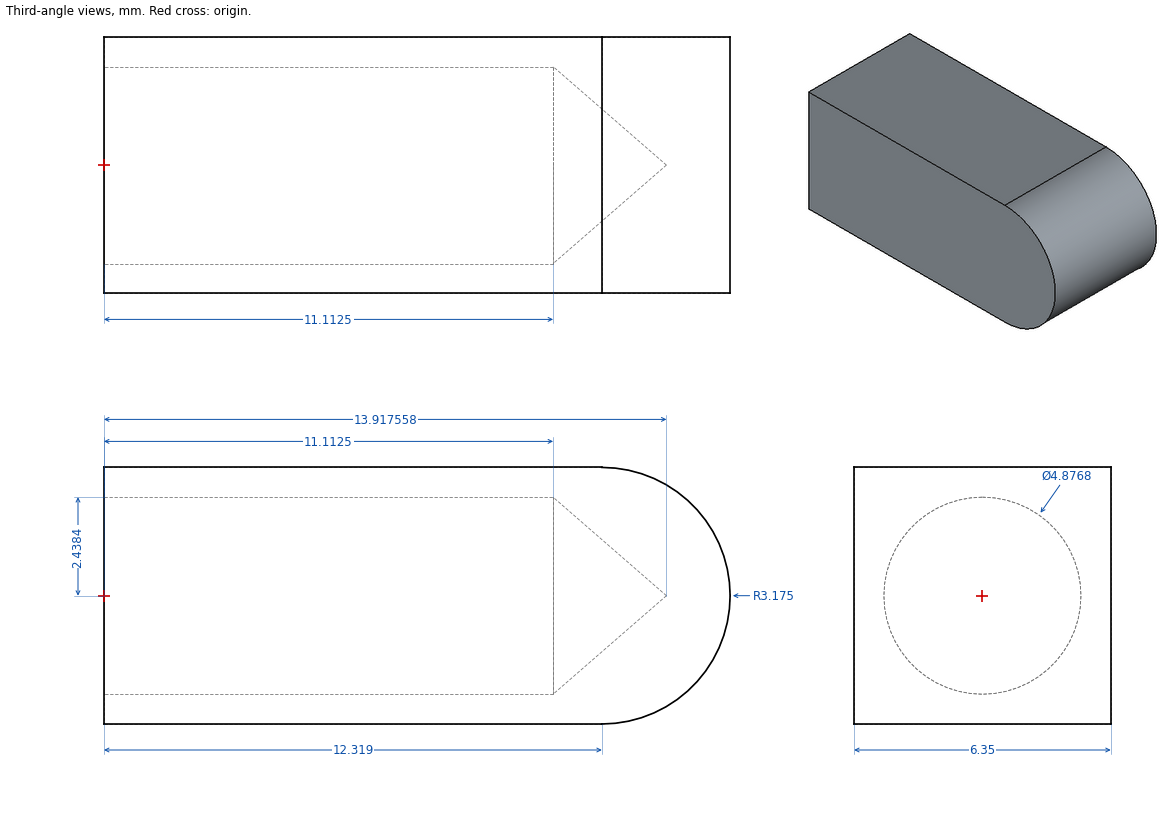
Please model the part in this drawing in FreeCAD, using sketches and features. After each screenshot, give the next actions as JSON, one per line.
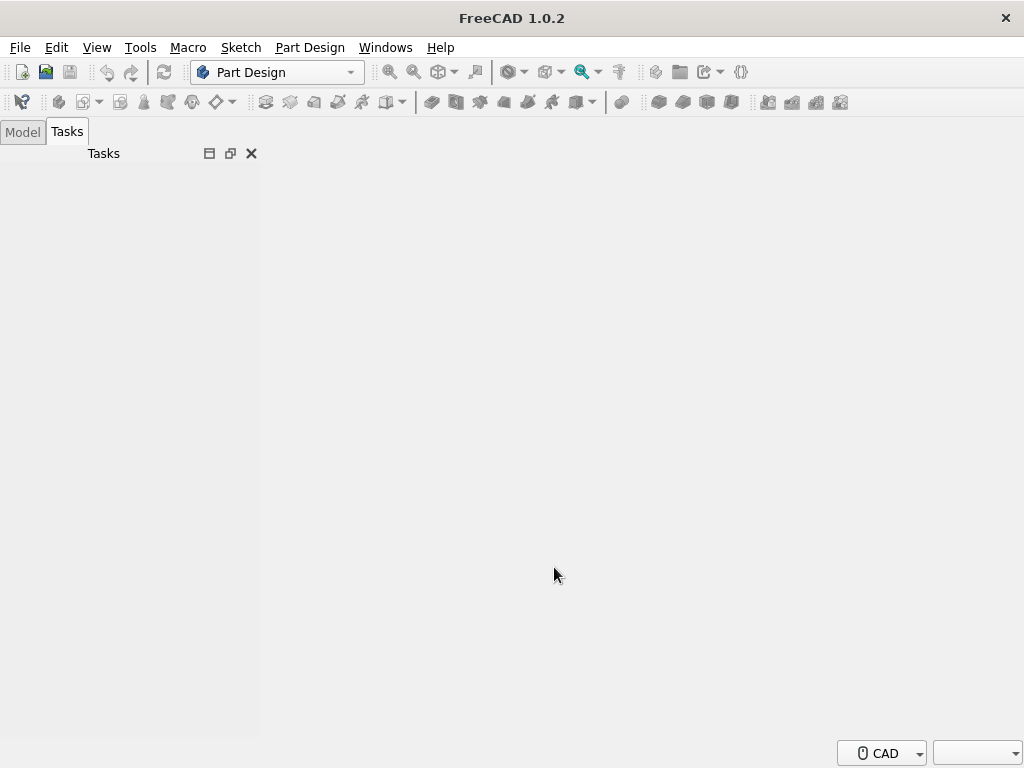
{"action": "key", "text": "ctrl+n"}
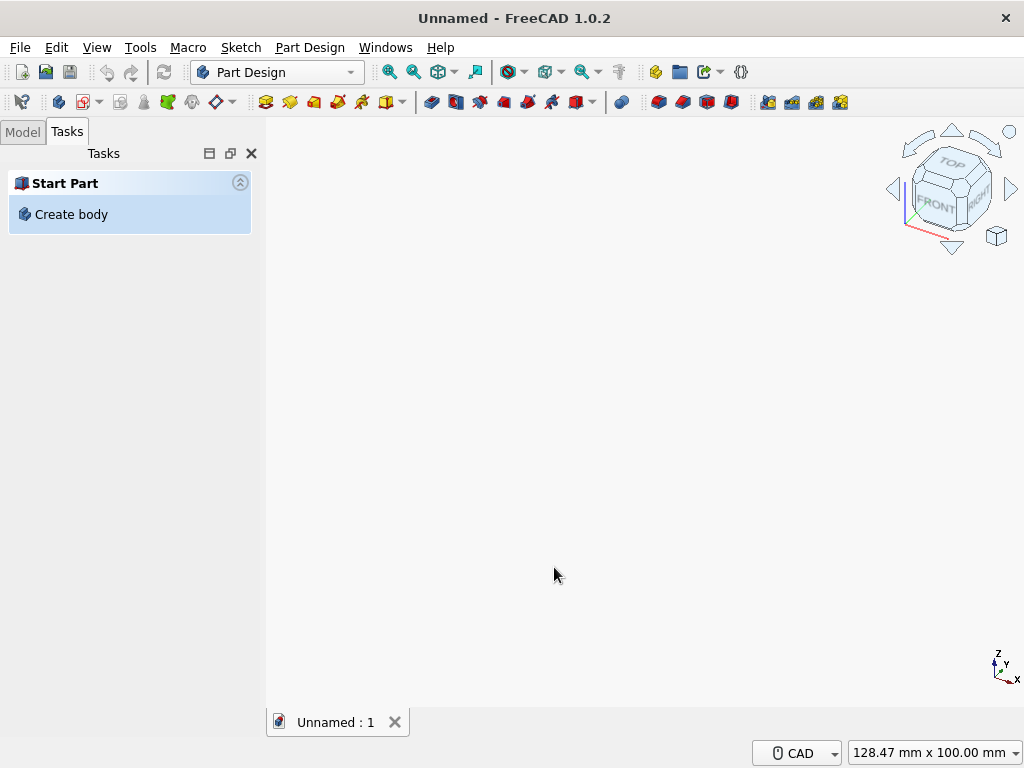
{"action": "left_click", "coordinate": [84, 102]}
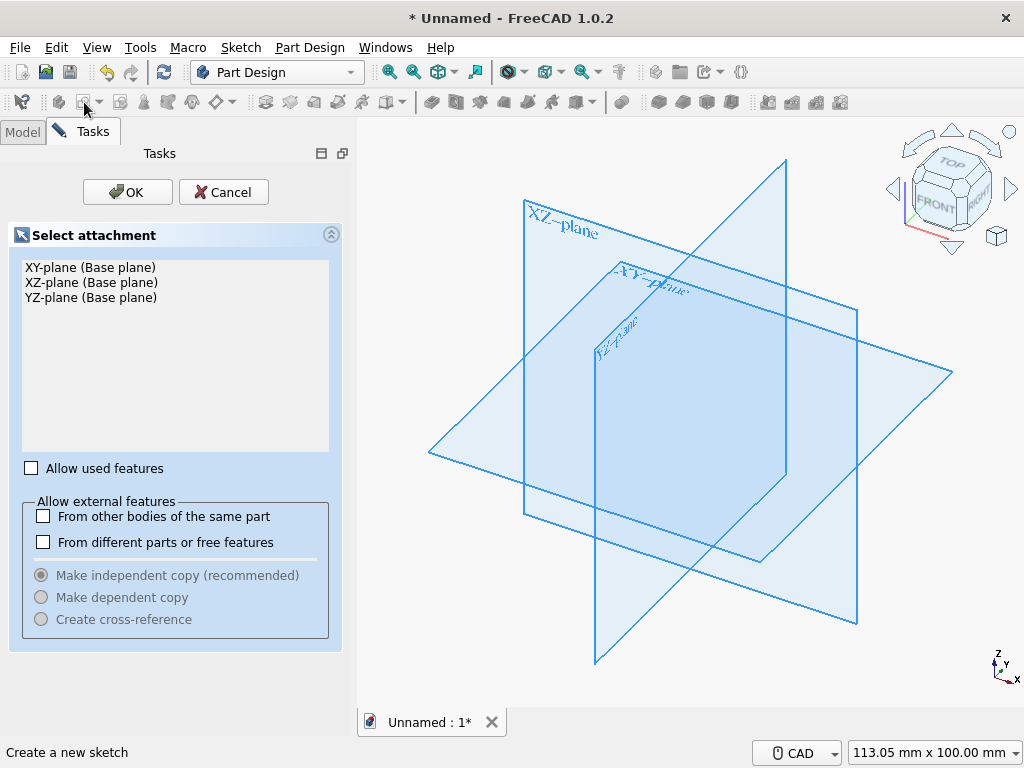
{"action": "left_click", "coordinate": [82, 282]}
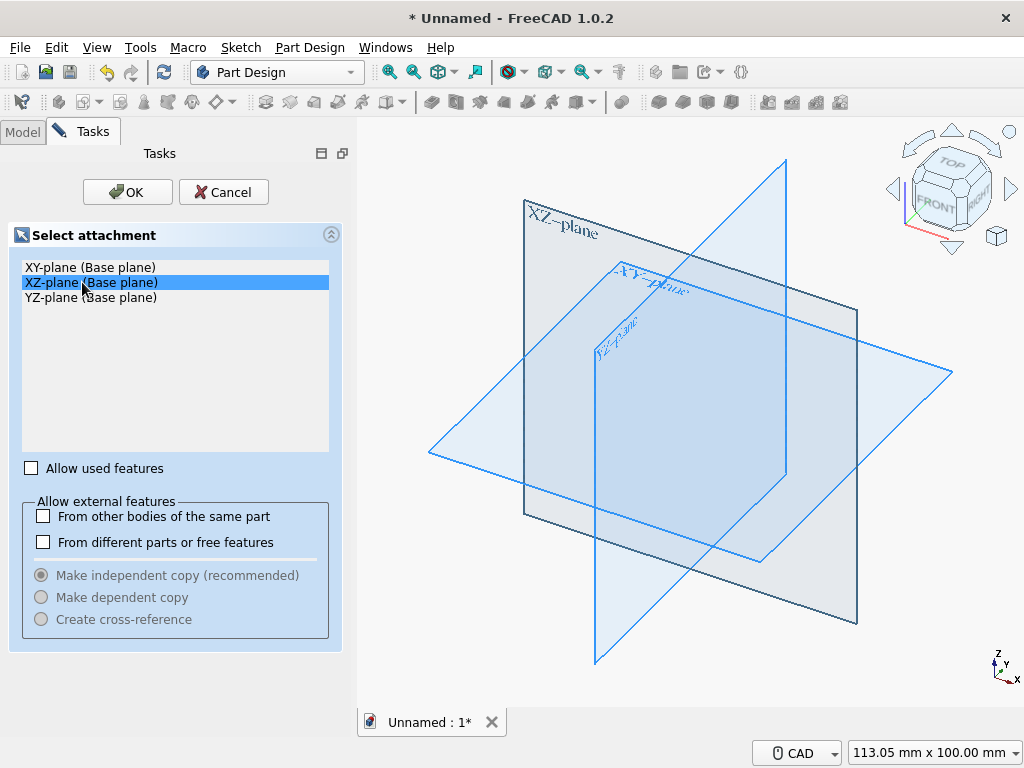
{"action": "left_click", "coordinate": [128, 192]}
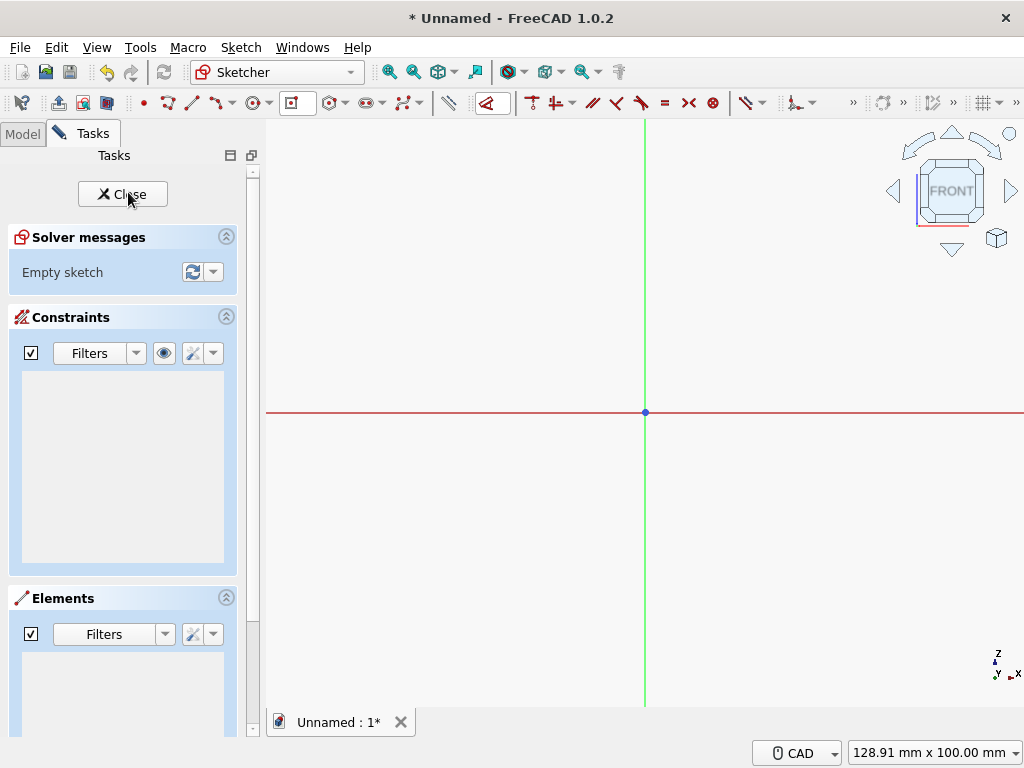
{"action": "scroll", "coordinate": [728, 413], "scroll_direction": "up", "scroll_amount": 7}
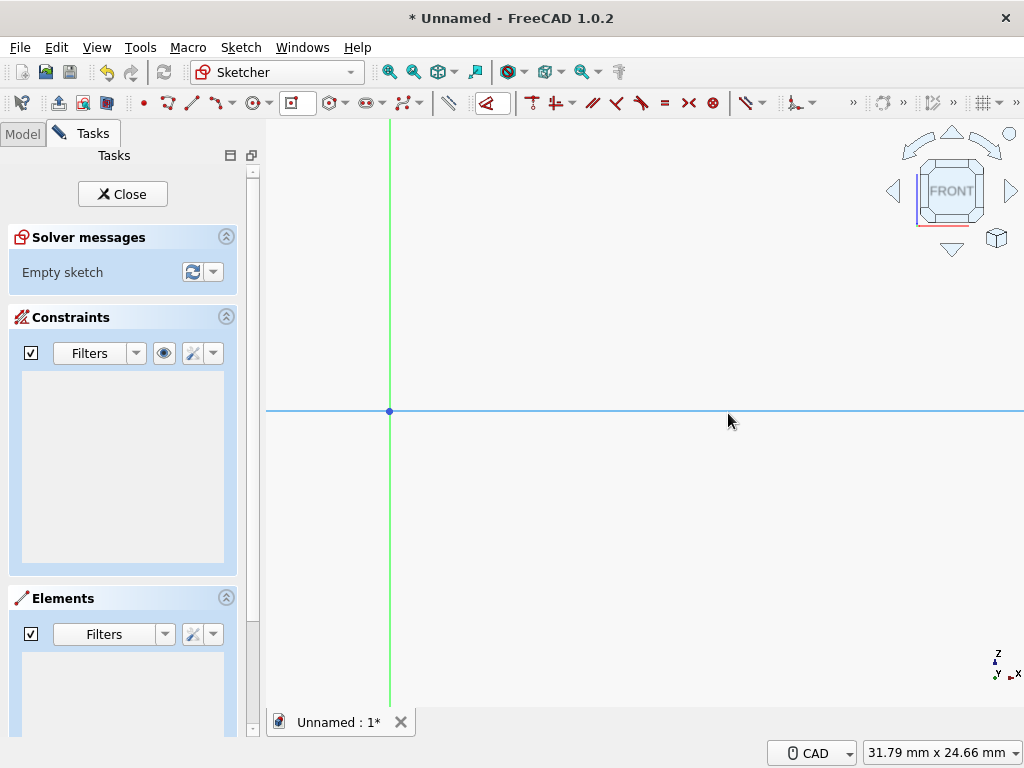
{"action": "left_click", "coordinate": [168, 104]}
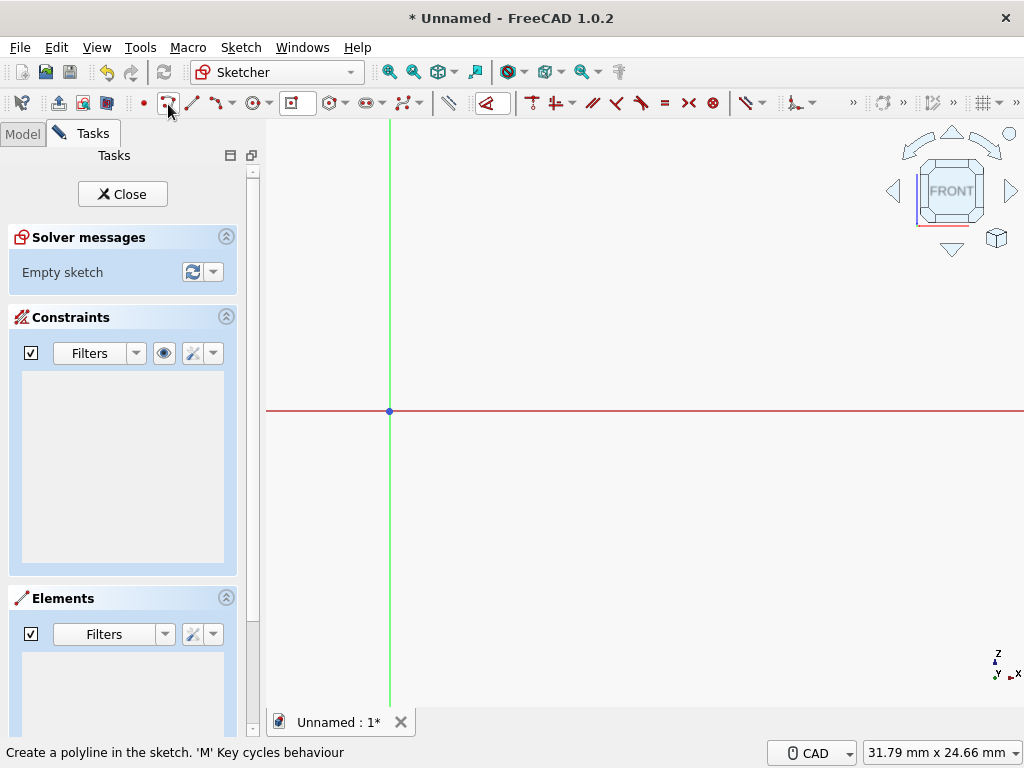
{"action": "left_click", "coordinate": [683, 487]}
{"action": "left_click", "coordinate": [390, 487]}
{"action": "left_click", "coordinate": [399, 336]}
{"action": "left_click", "coordinate": [683, 336]}
{"action": "right_click", "coordinate": [683, 336]}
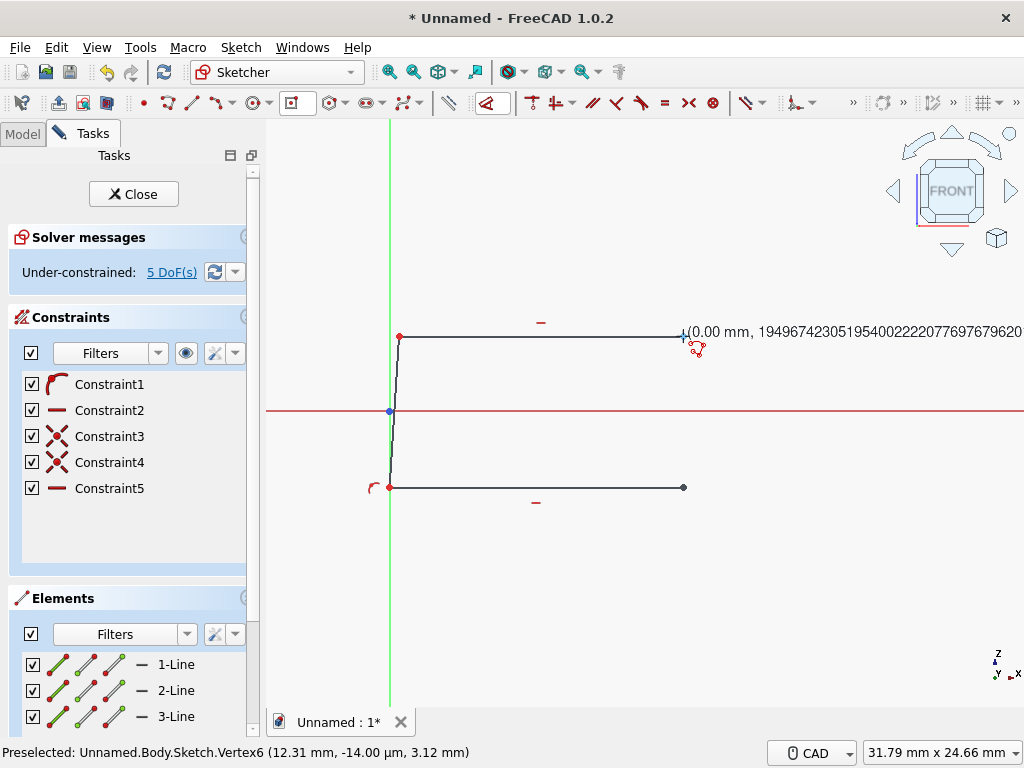
{"action": "key", "text": "g 3 a"}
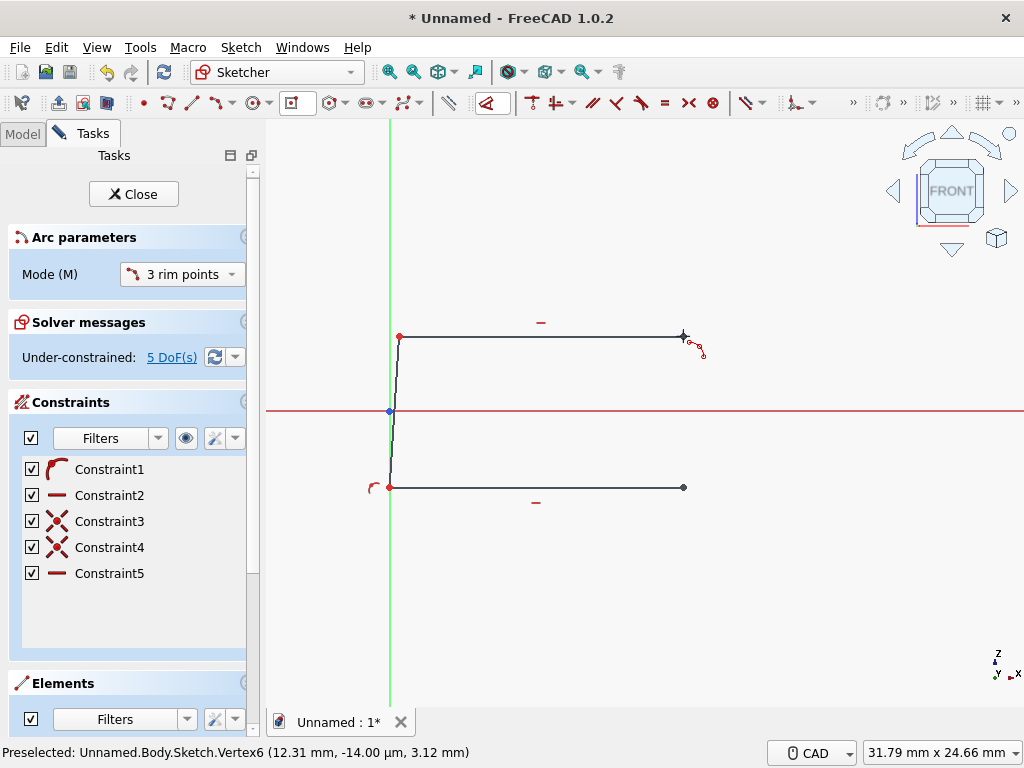
{"action": "left_click", "coordinate": [683, 337]}
{"action": "left_click", "coordinate": [683, 488]}
{"action": "left_click", "coordinate": [755, 435]}
{"action": "key", "text": "Escape"}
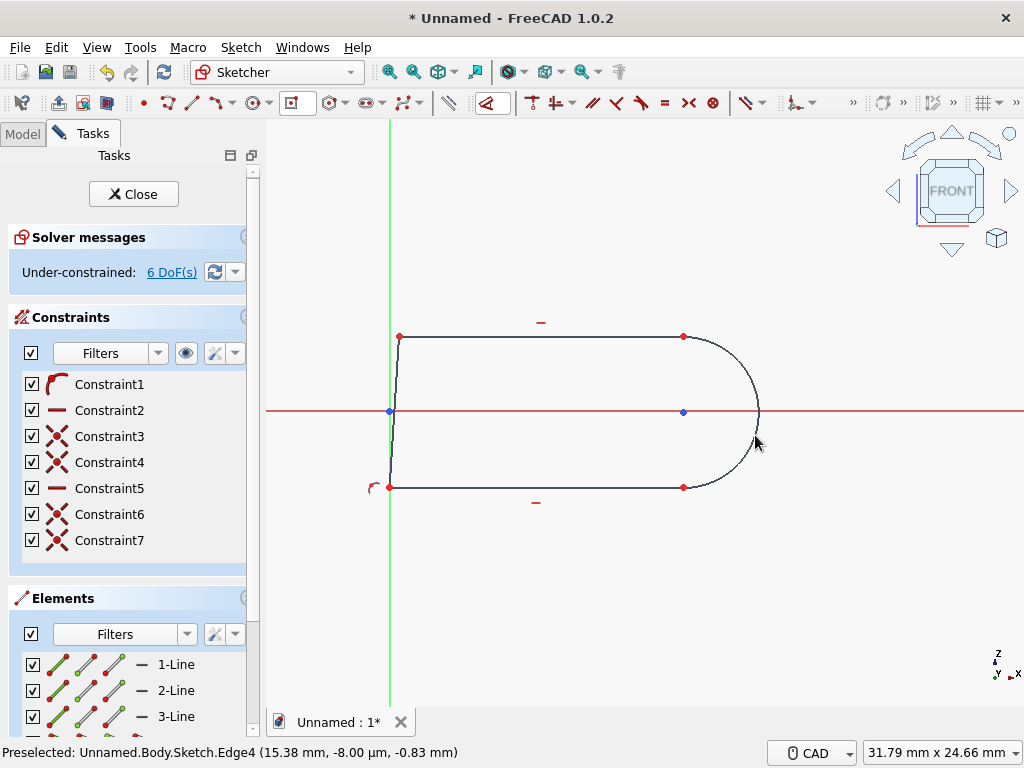
{"action": "left_click", "coordinate": [595, 488]}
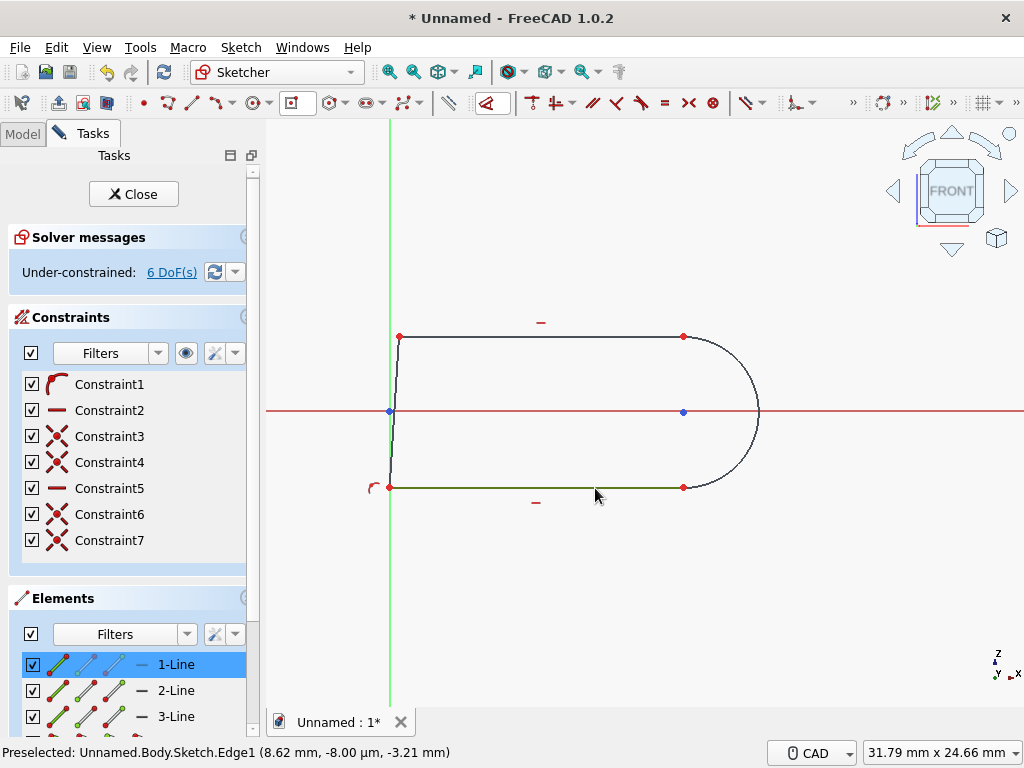
{"action": "left_click", "coordinate": [744, 457]}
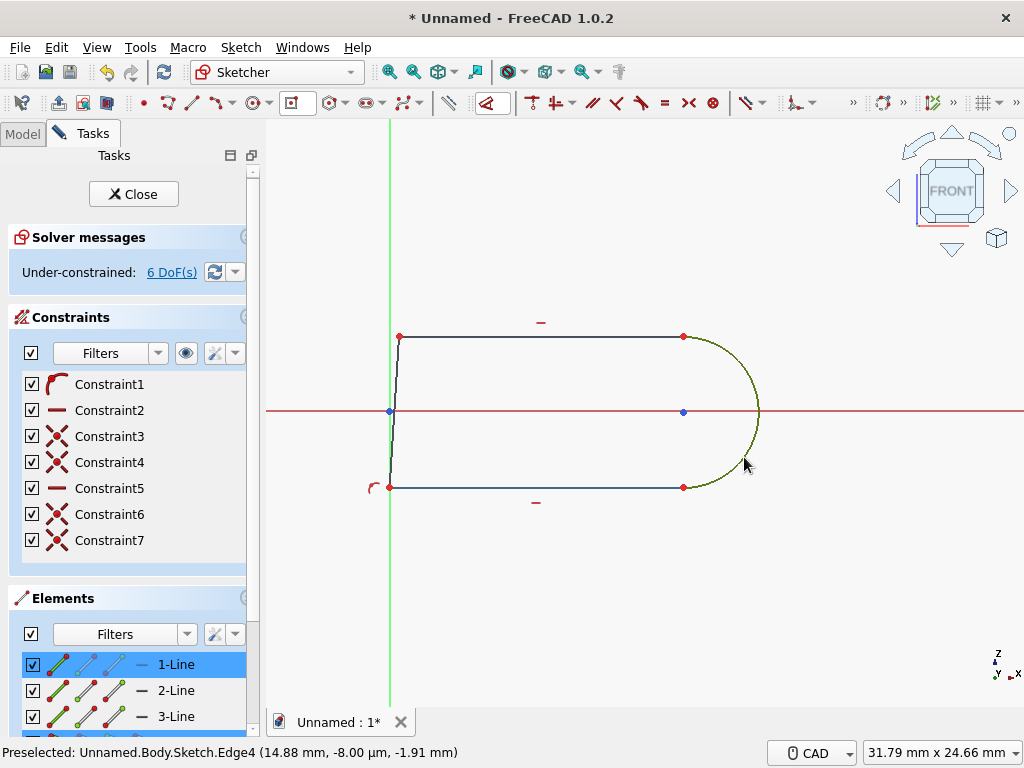
{"action": "left_click", "coordinate": [642, 104]}